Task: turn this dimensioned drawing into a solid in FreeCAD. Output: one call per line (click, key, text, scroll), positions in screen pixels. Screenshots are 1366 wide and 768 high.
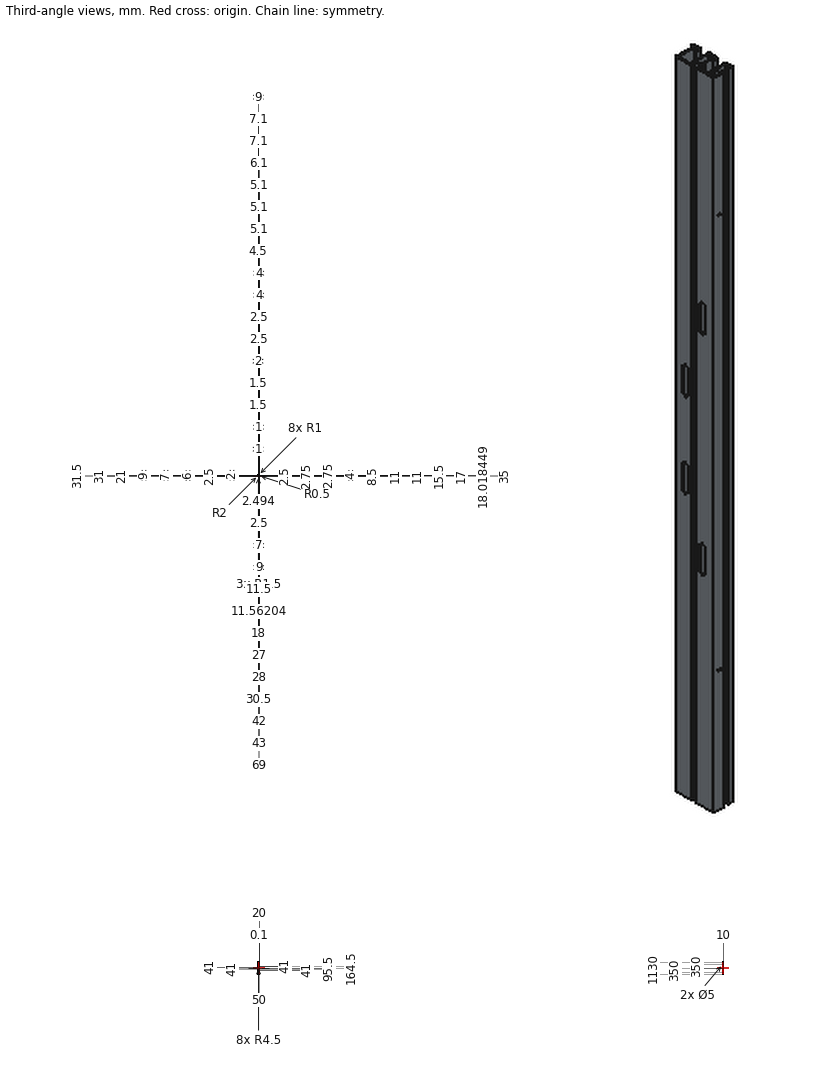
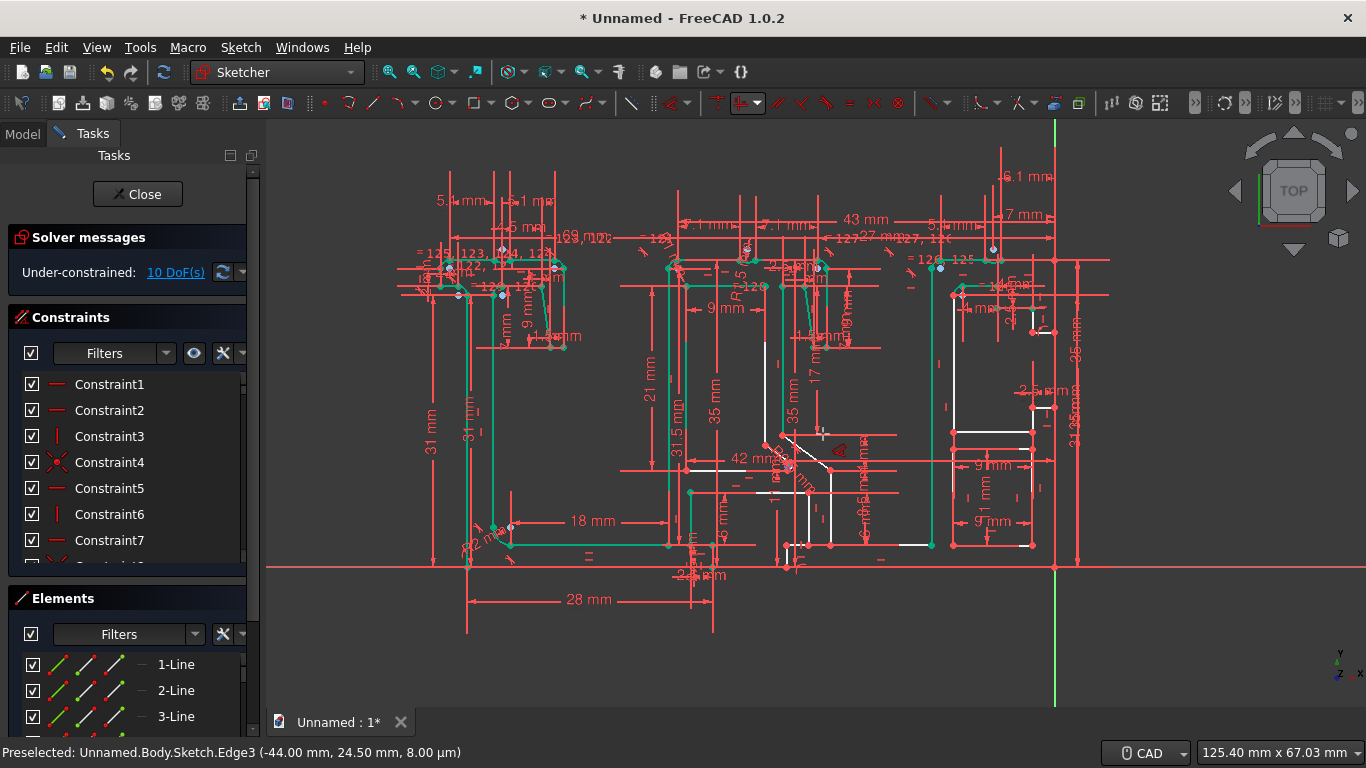
click(867, 567)
click(921, 601)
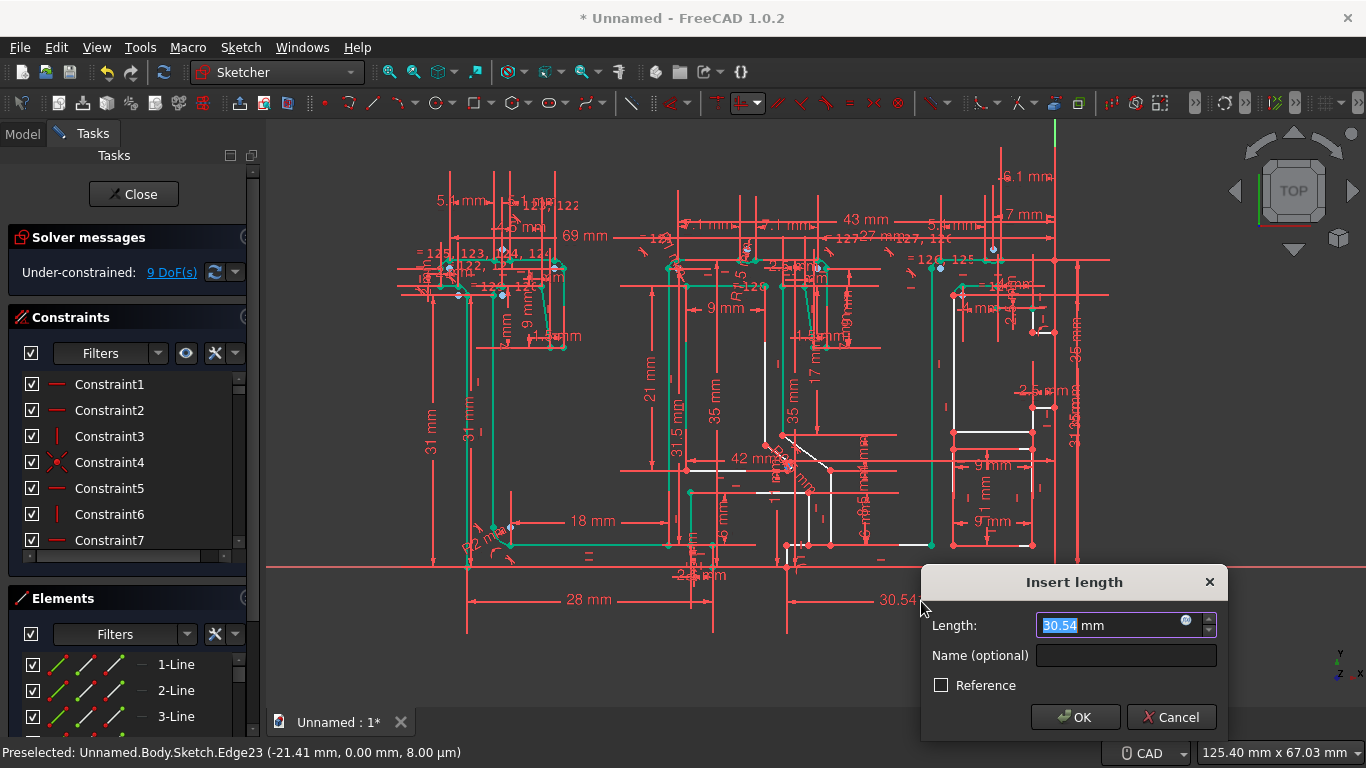
text(30.5)
key(Return)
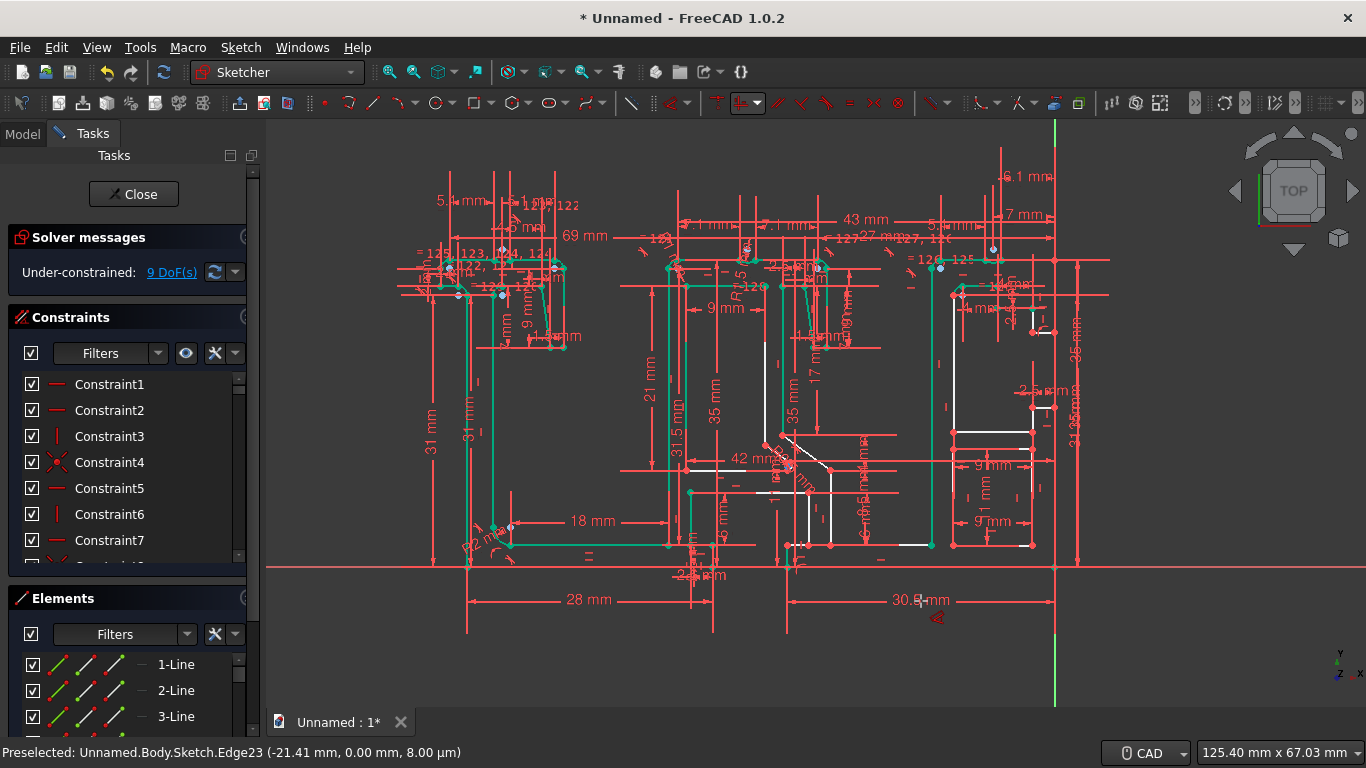
scroll(1033, 417, up, 3)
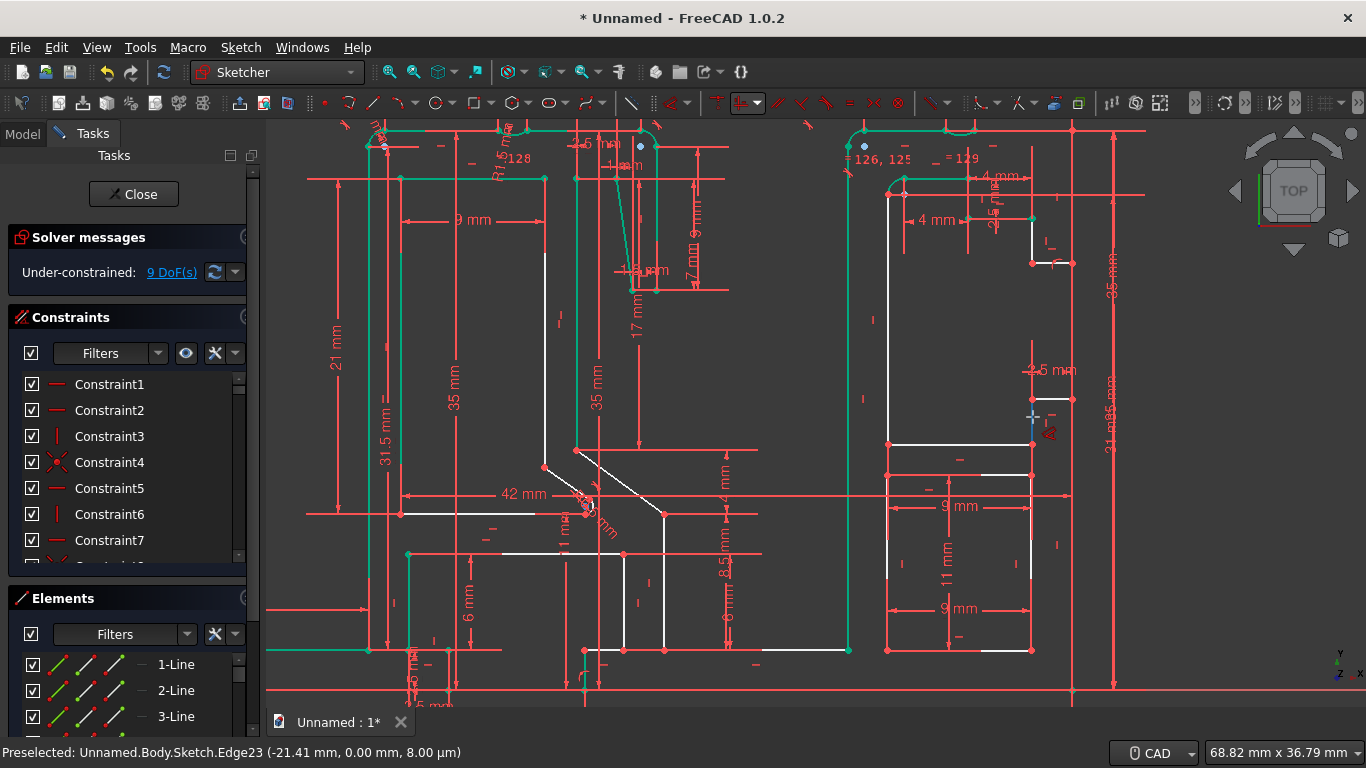
click(1032, 417)
click(998, 422)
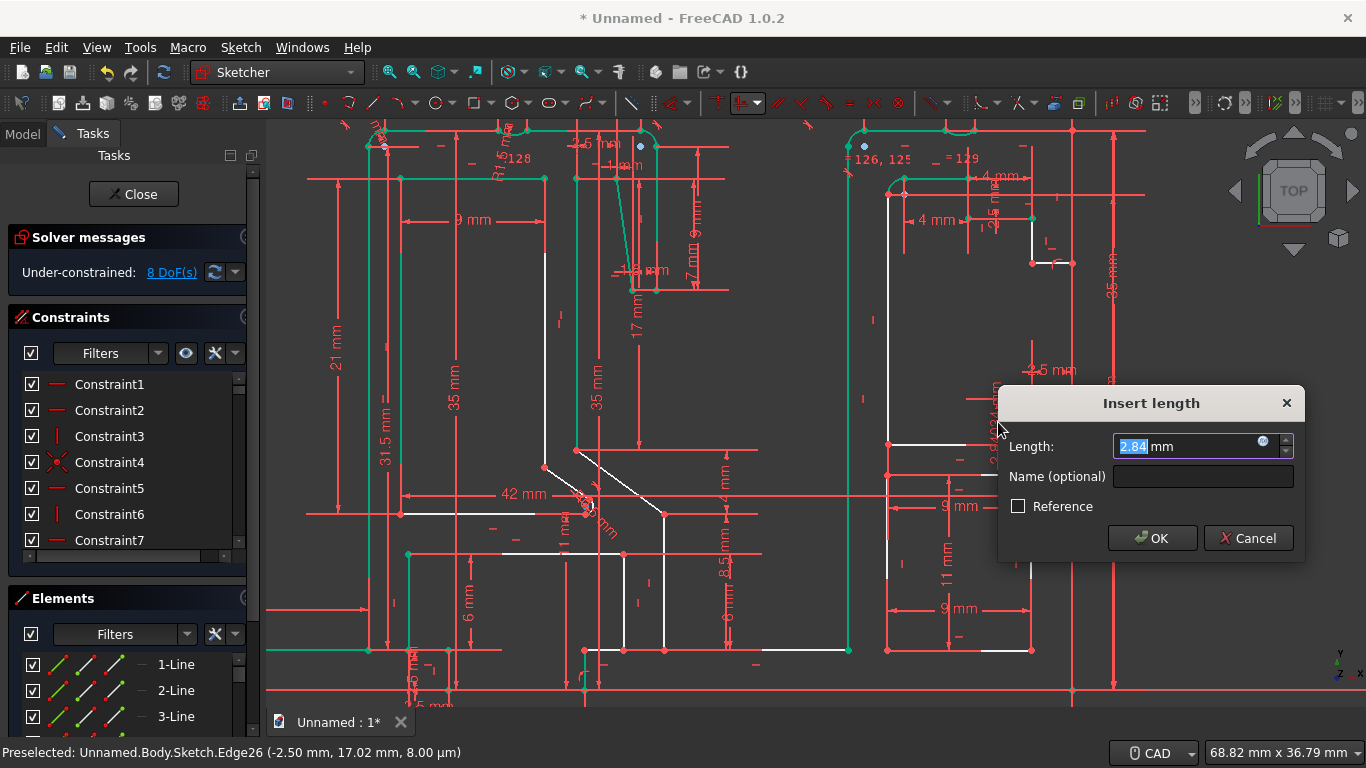
text(2.75)
key(Return)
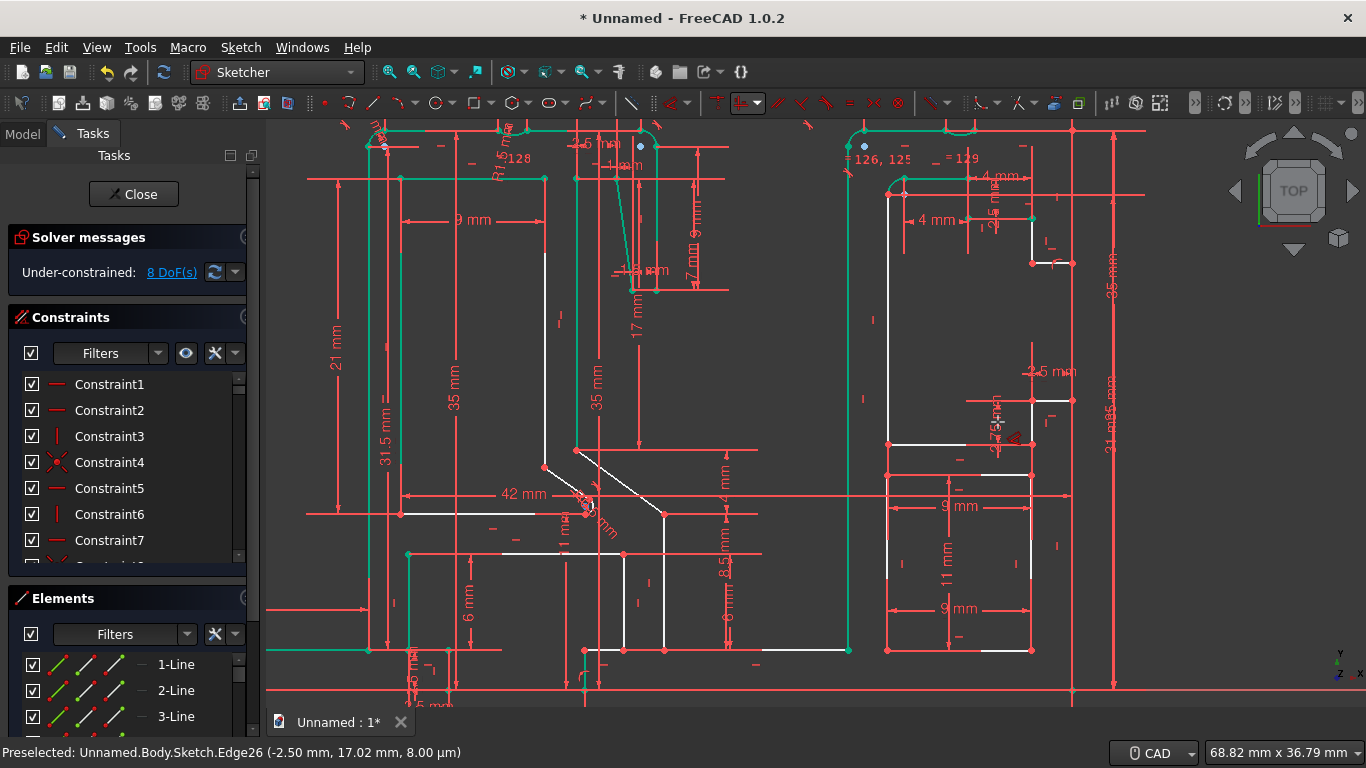
click(888, 370)
click(922, 320)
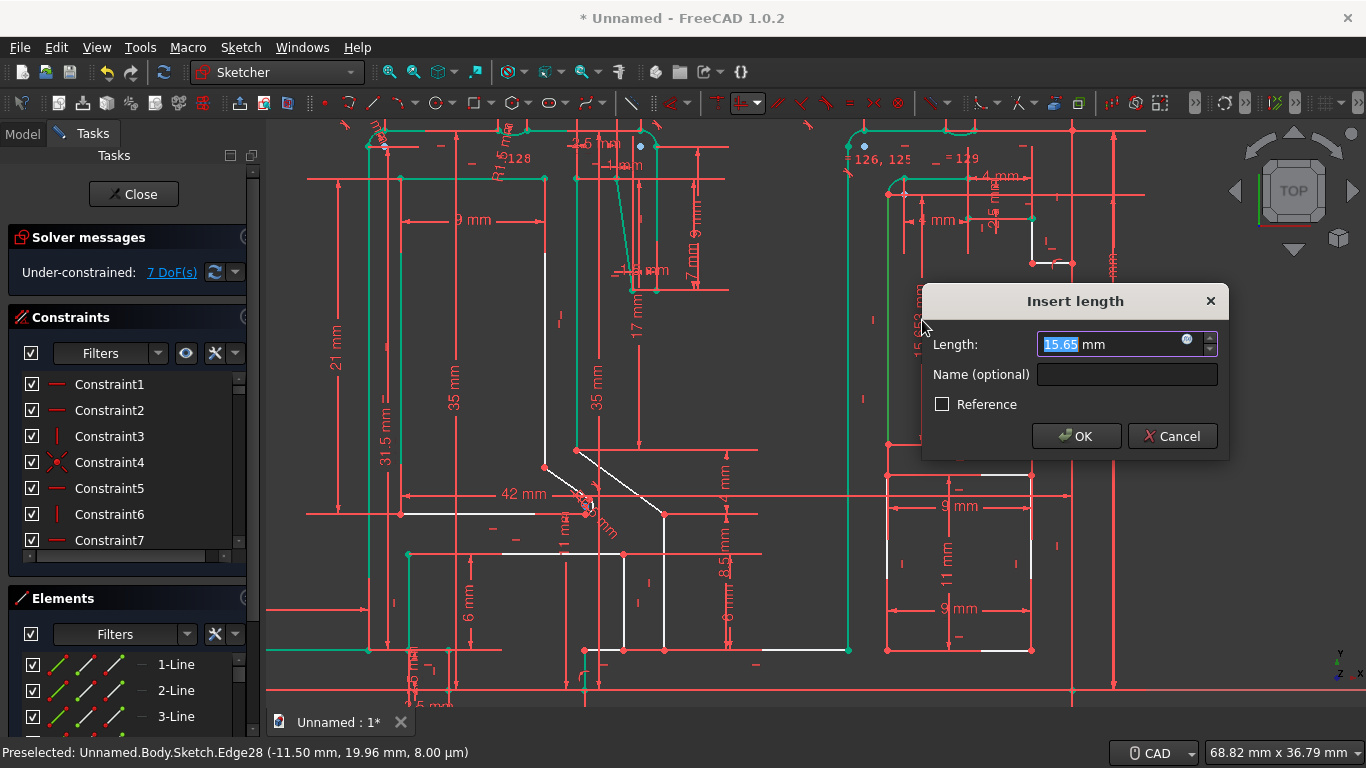
text(15.5)
key(Return)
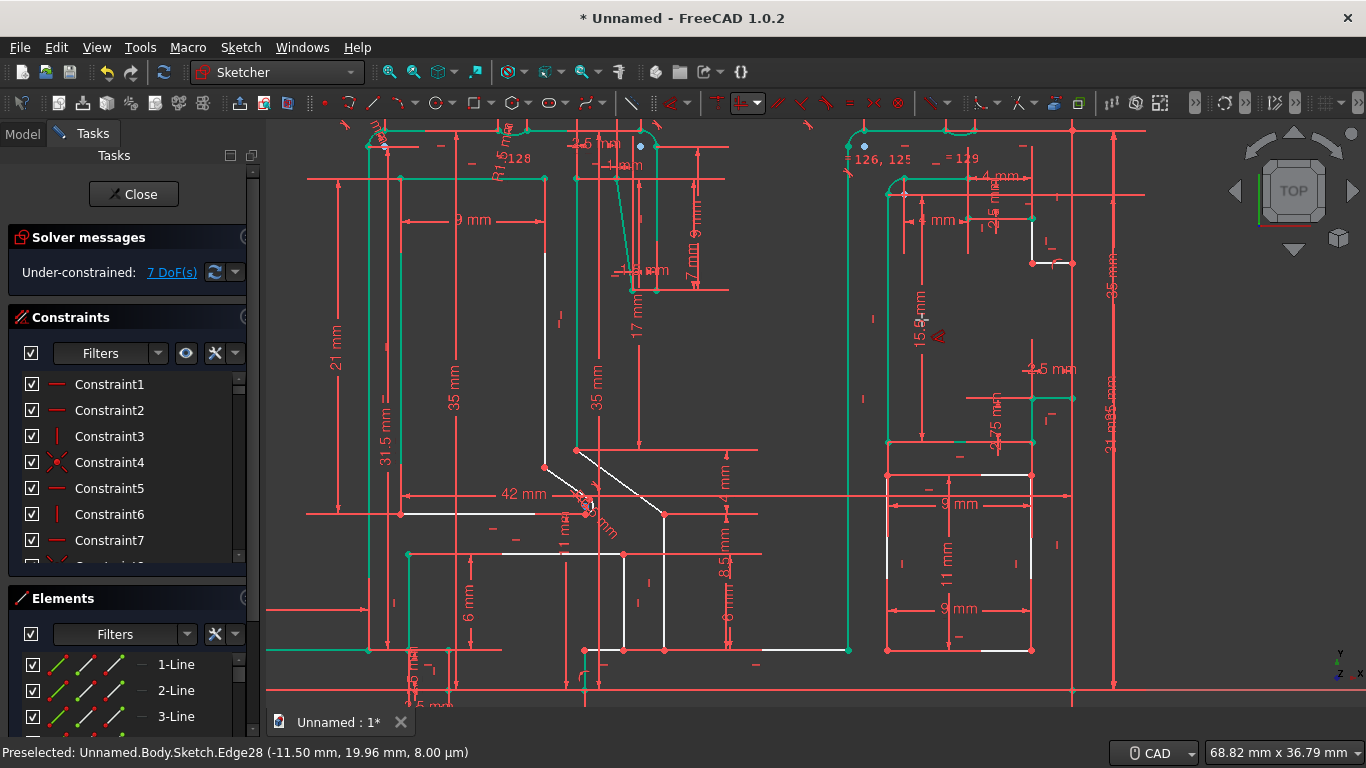
click(1032, 232)
click(998, 241)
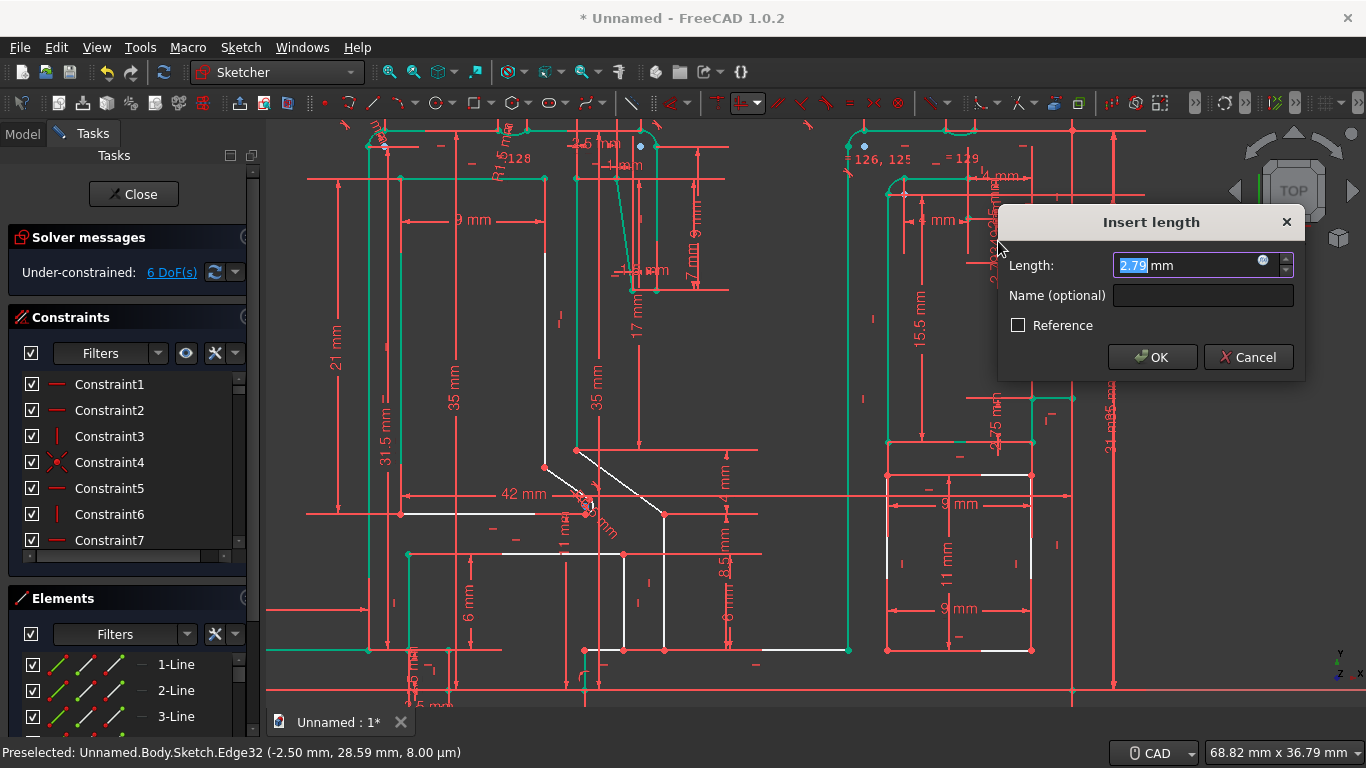
text(2.75)
key(Return)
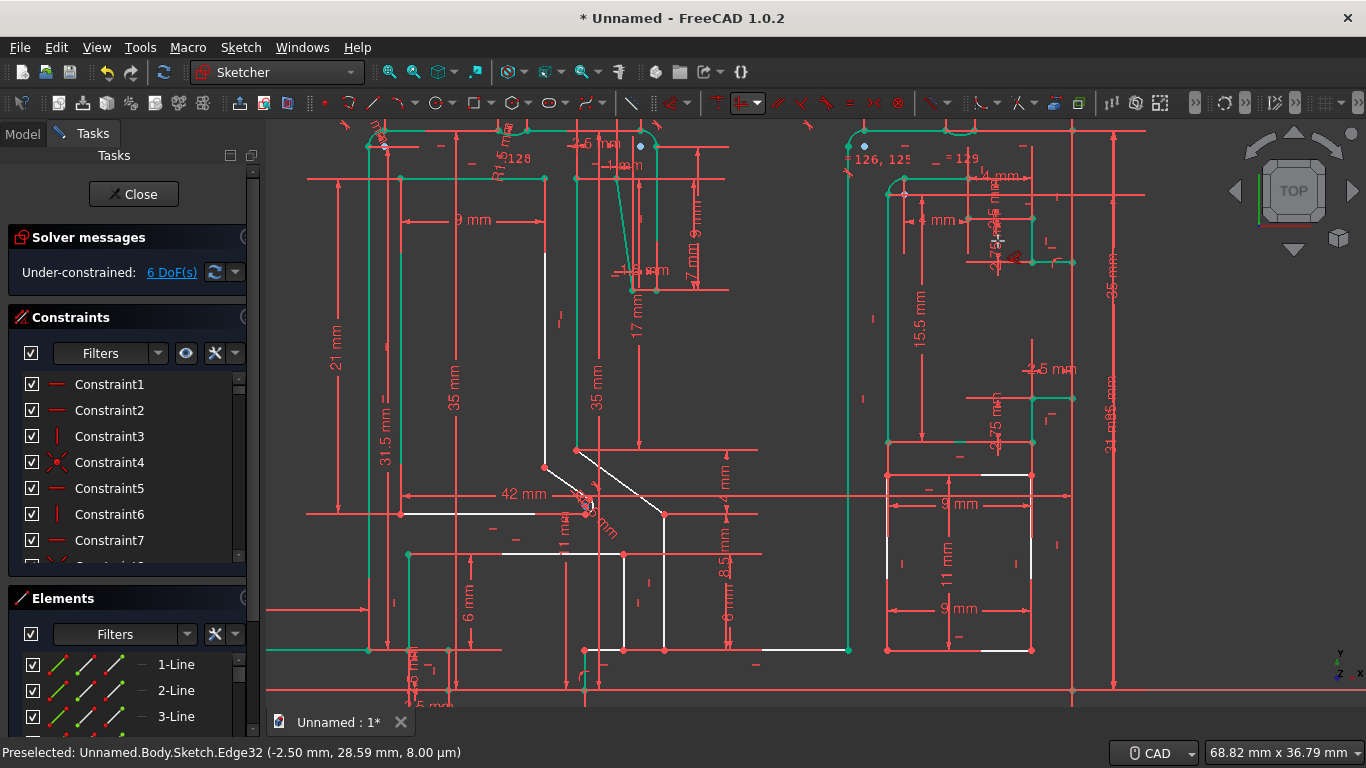
click(793, 650)
click(821, 616)